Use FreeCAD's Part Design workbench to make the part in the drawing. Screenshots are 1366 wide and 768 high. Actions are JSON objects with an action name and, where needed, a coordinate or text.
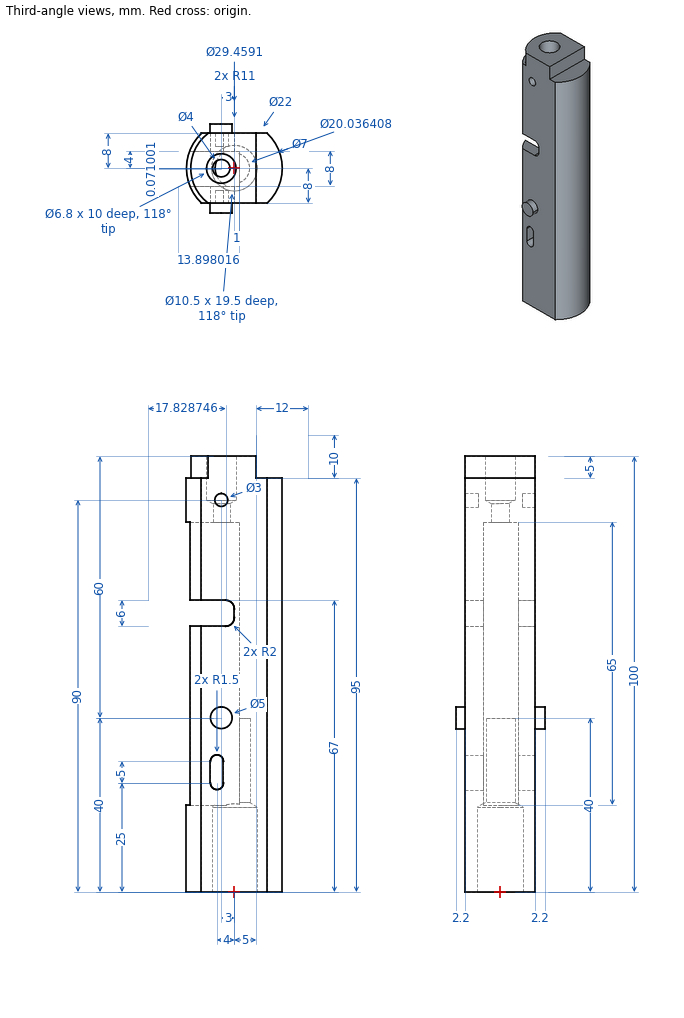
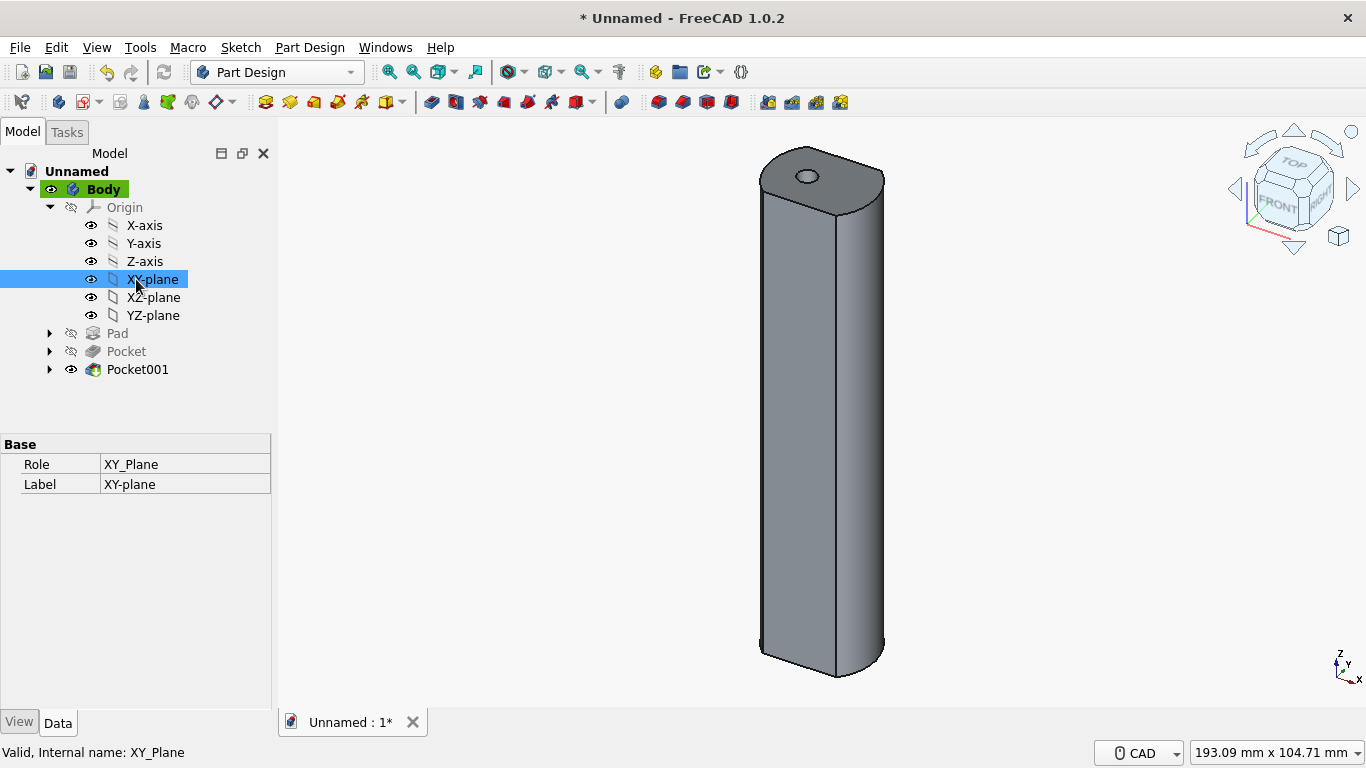
{"action": "left_click", "coordinate": [216, 102]}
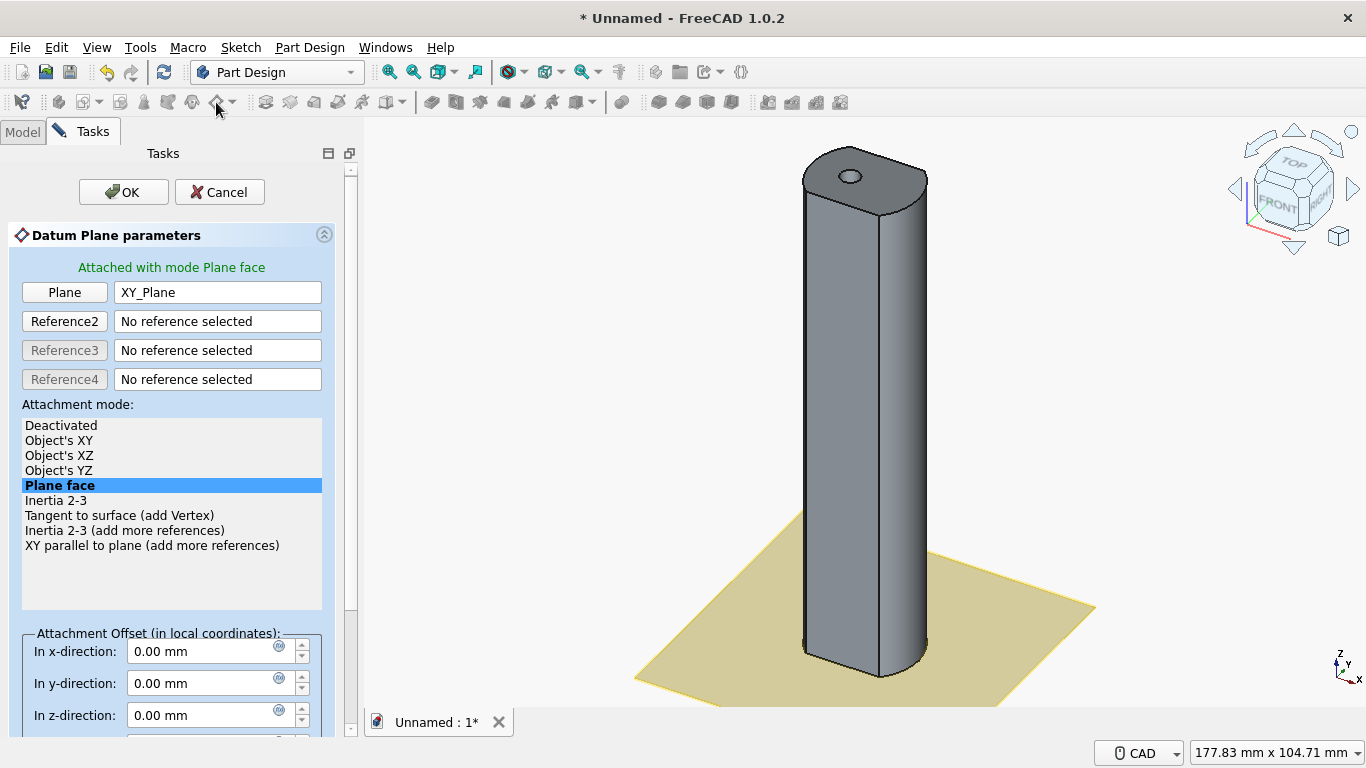
{"action": "triple_click", "coordinate": [210, 715]}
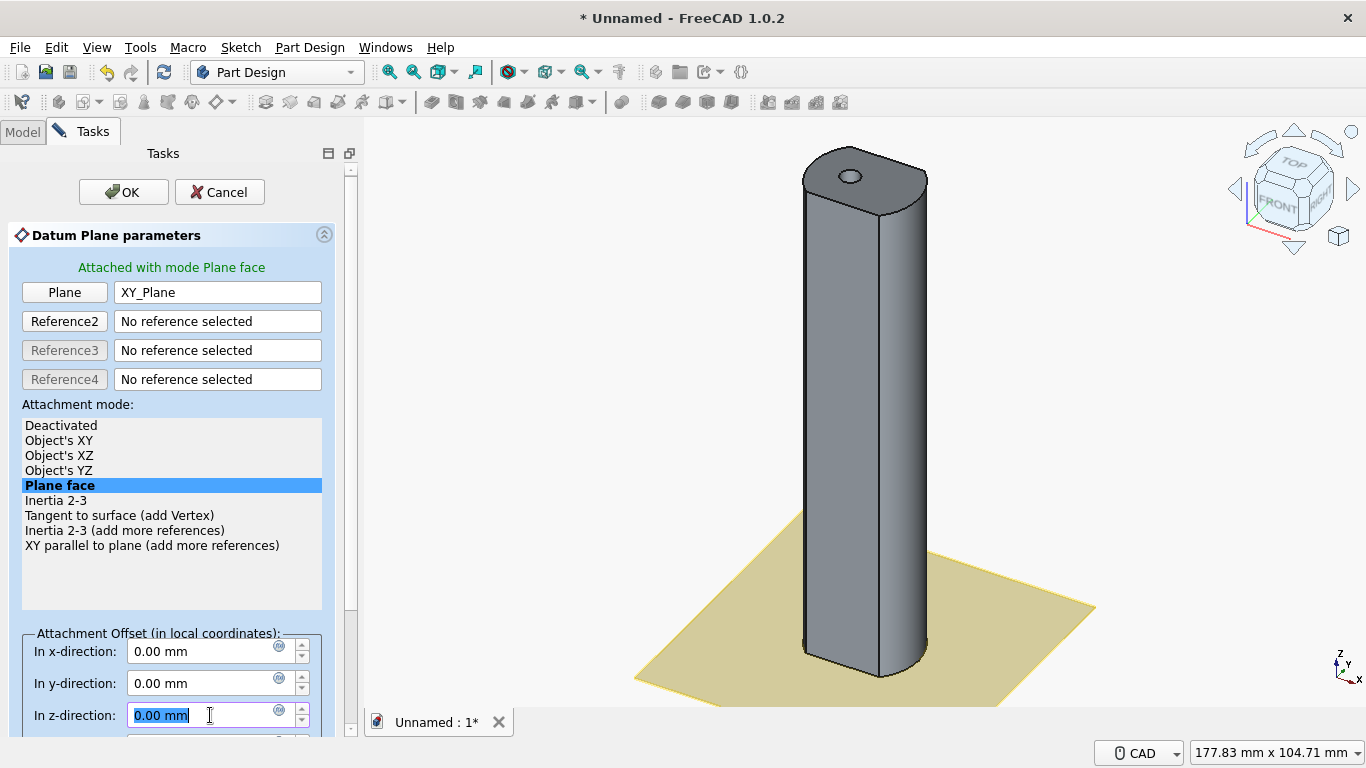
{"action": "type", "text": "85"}
{"action": "key", "text": "Tab"}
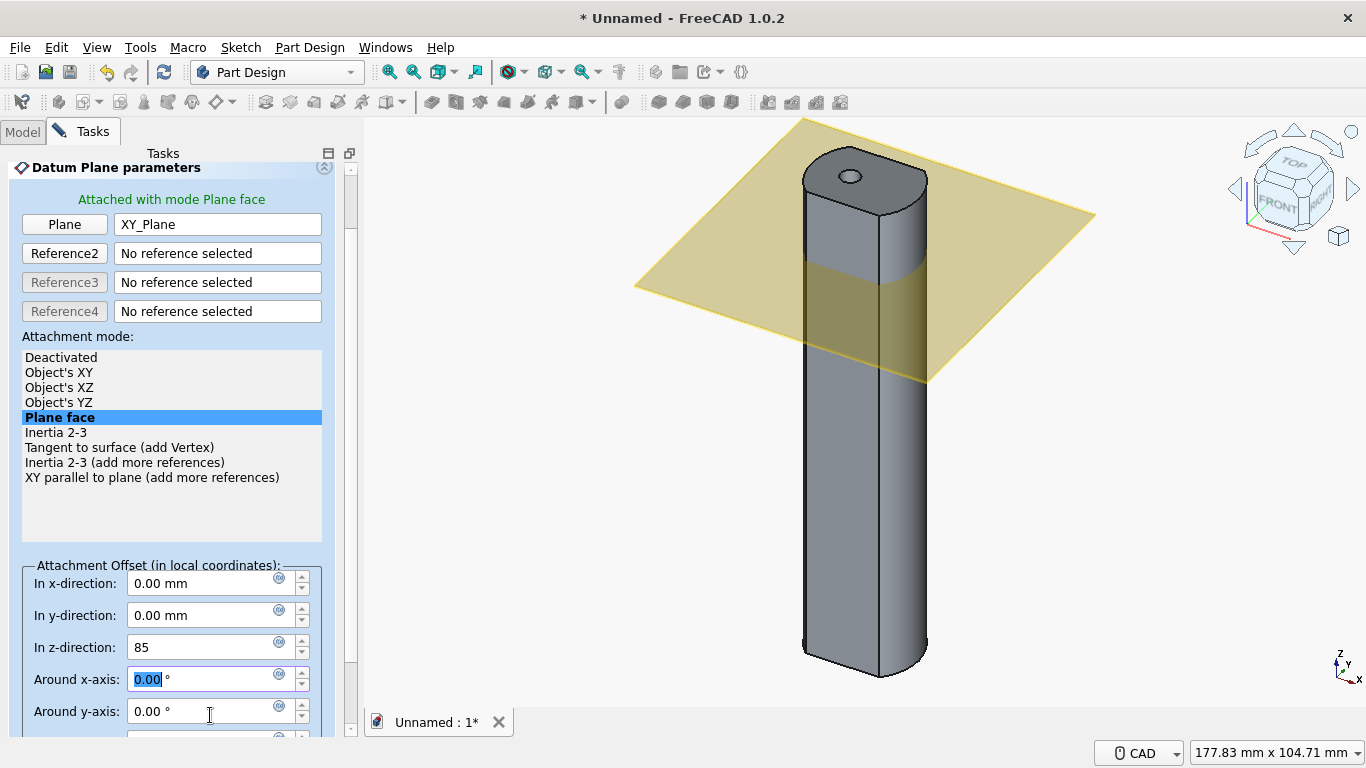
{"action": "scroll", "coordinate": [351, 450], "scroll_direction": "up", "scroll_amount": 2}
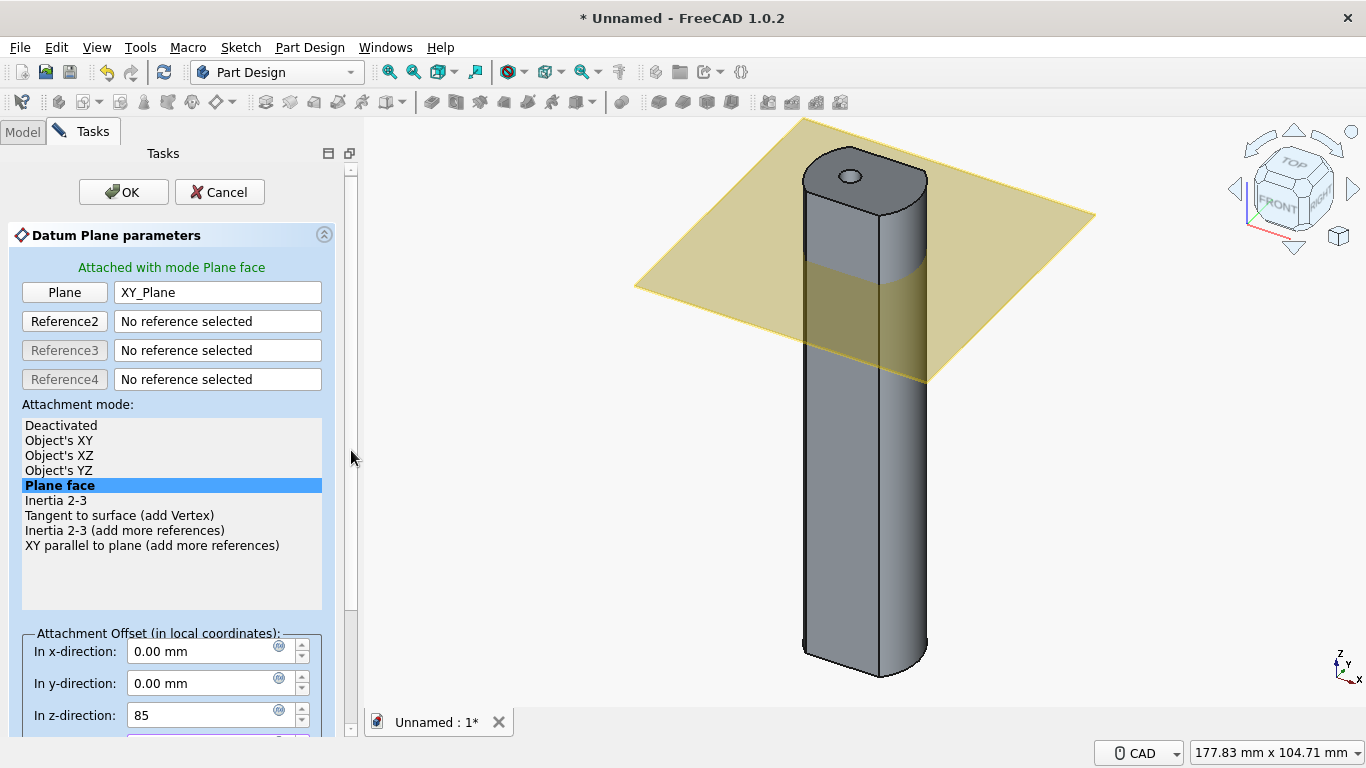
{"action": "left_click", "coordinate": [124, 192]}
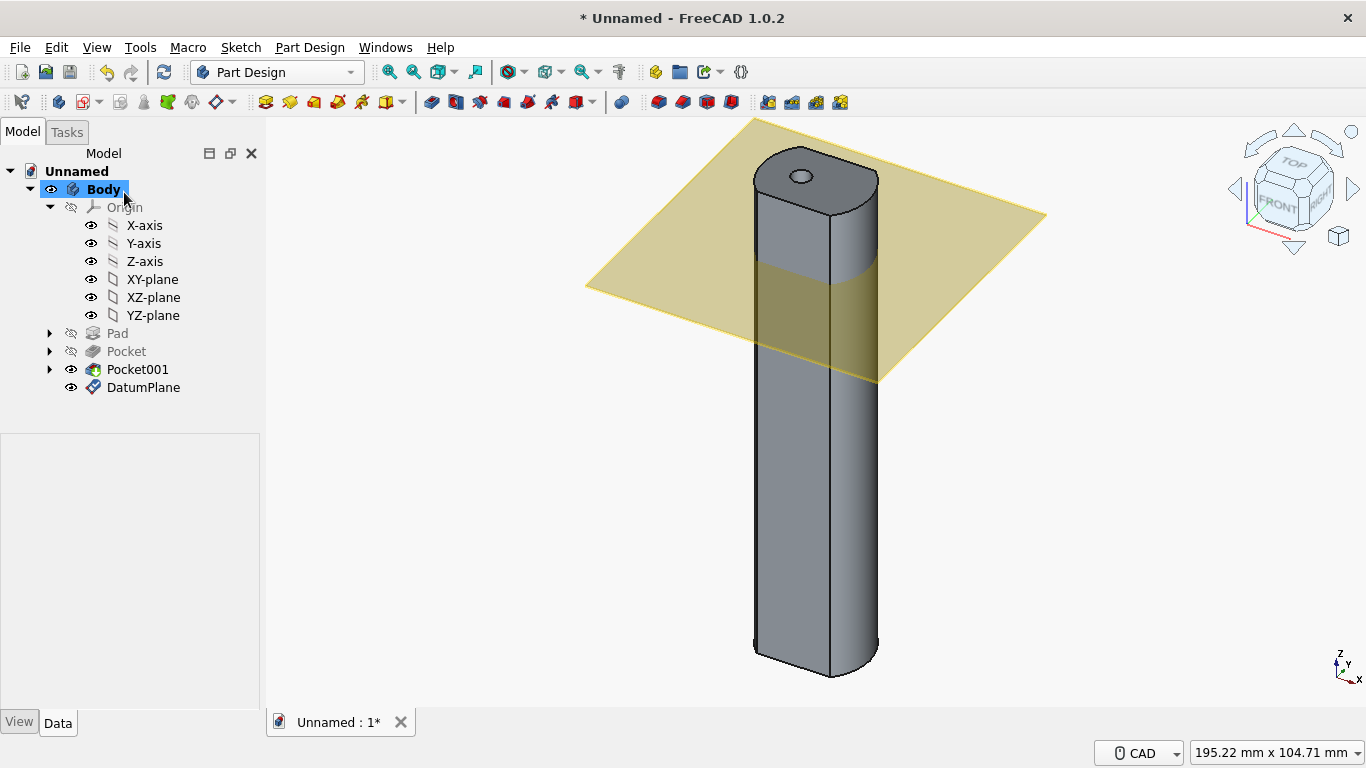
{"action": "left_click", "coordinate": [116, 387]}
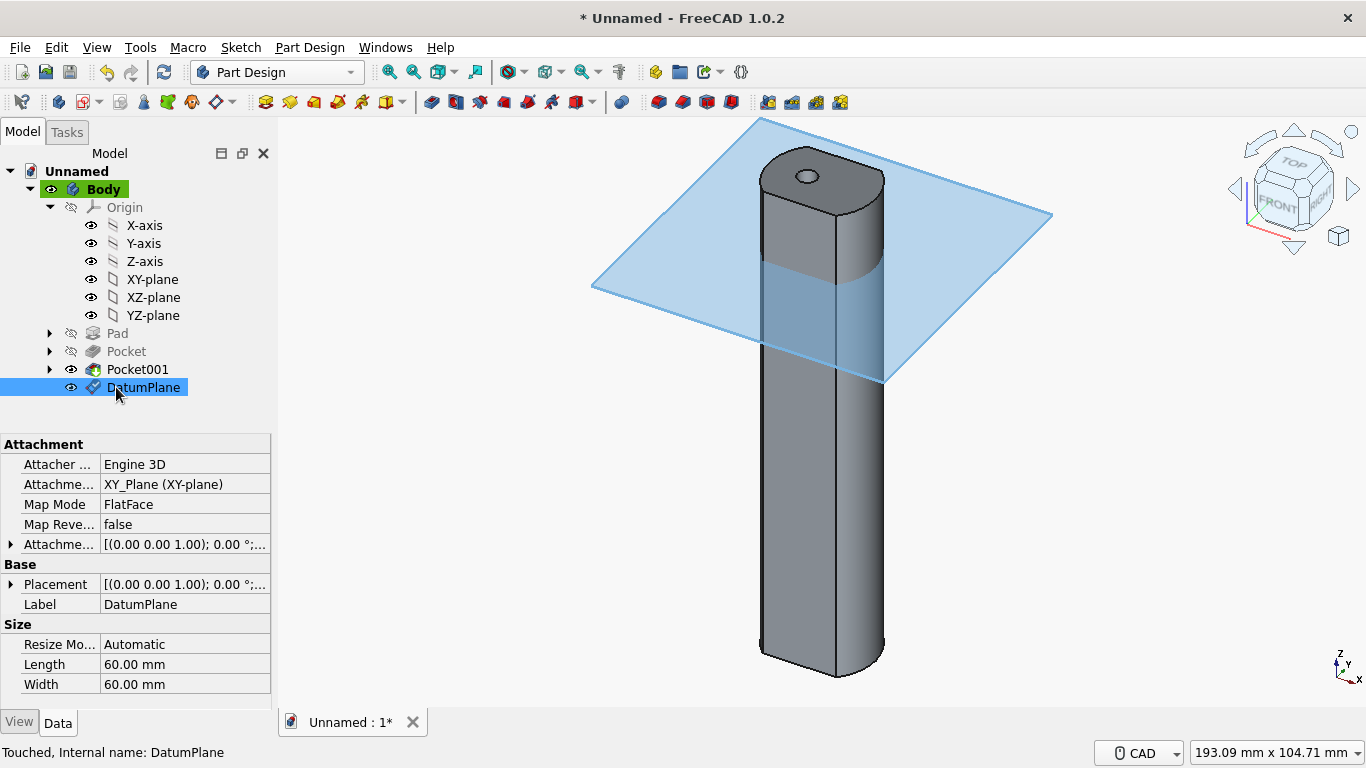
{"action": "left_click", "coordinate": [84, 102]}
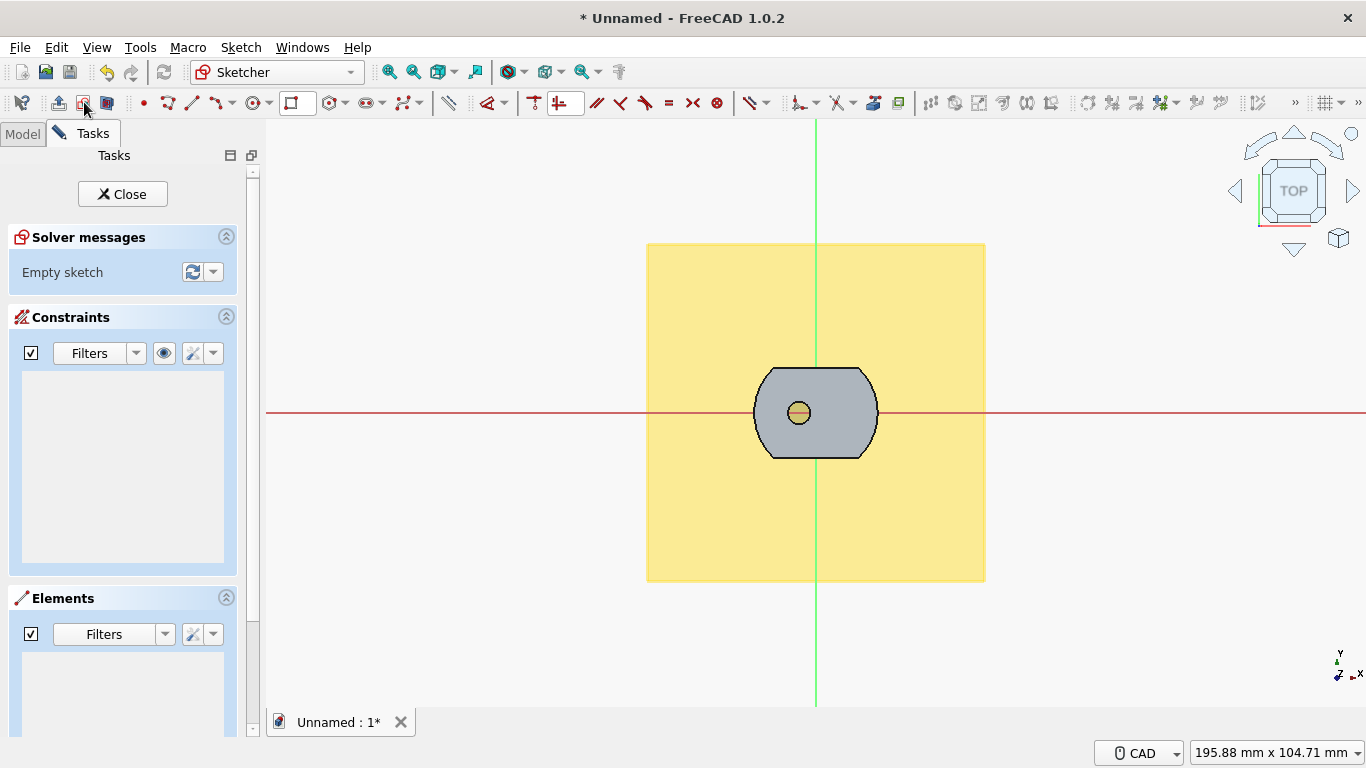
{"action": "left_click", "coordinate": [108, 104]}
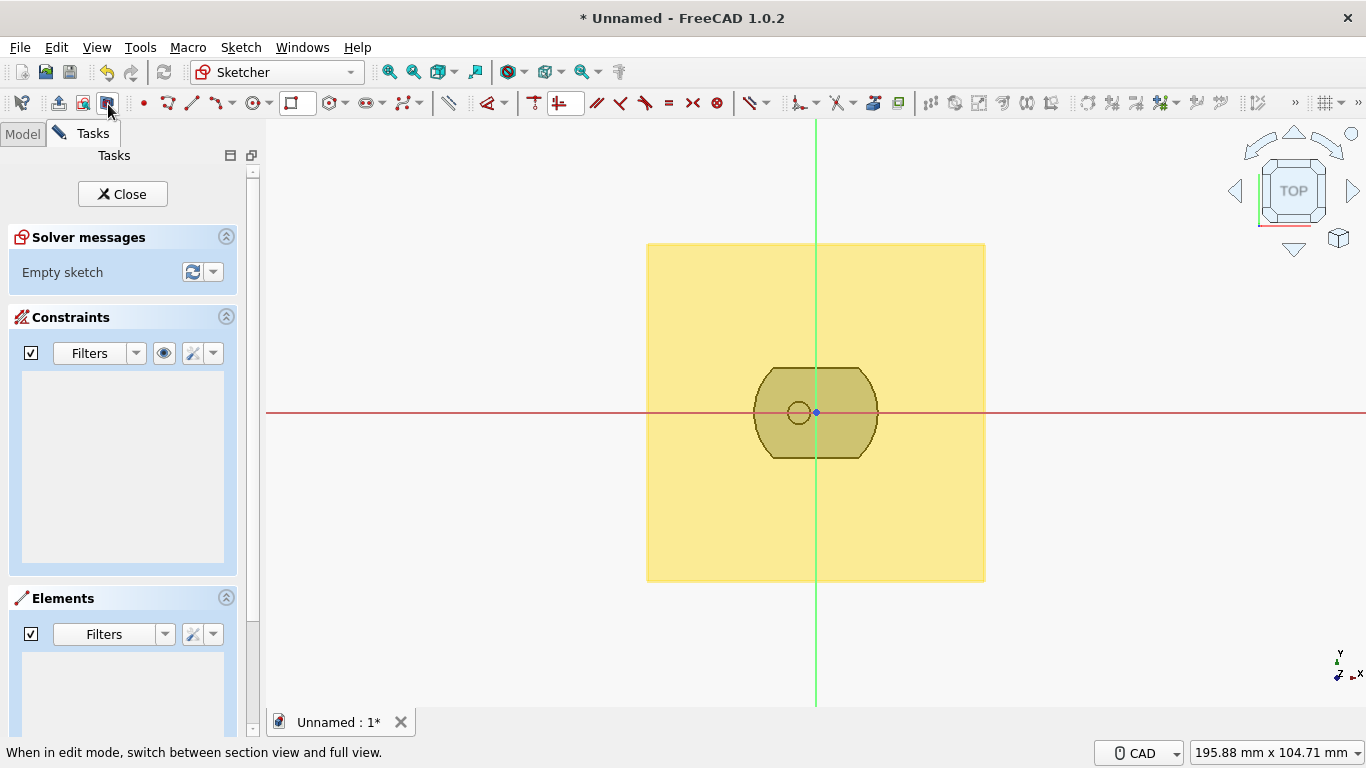
{"action": "scroll", "coordinate": [787, 413], "scroll_direction": "up", "scroll_amount": 11}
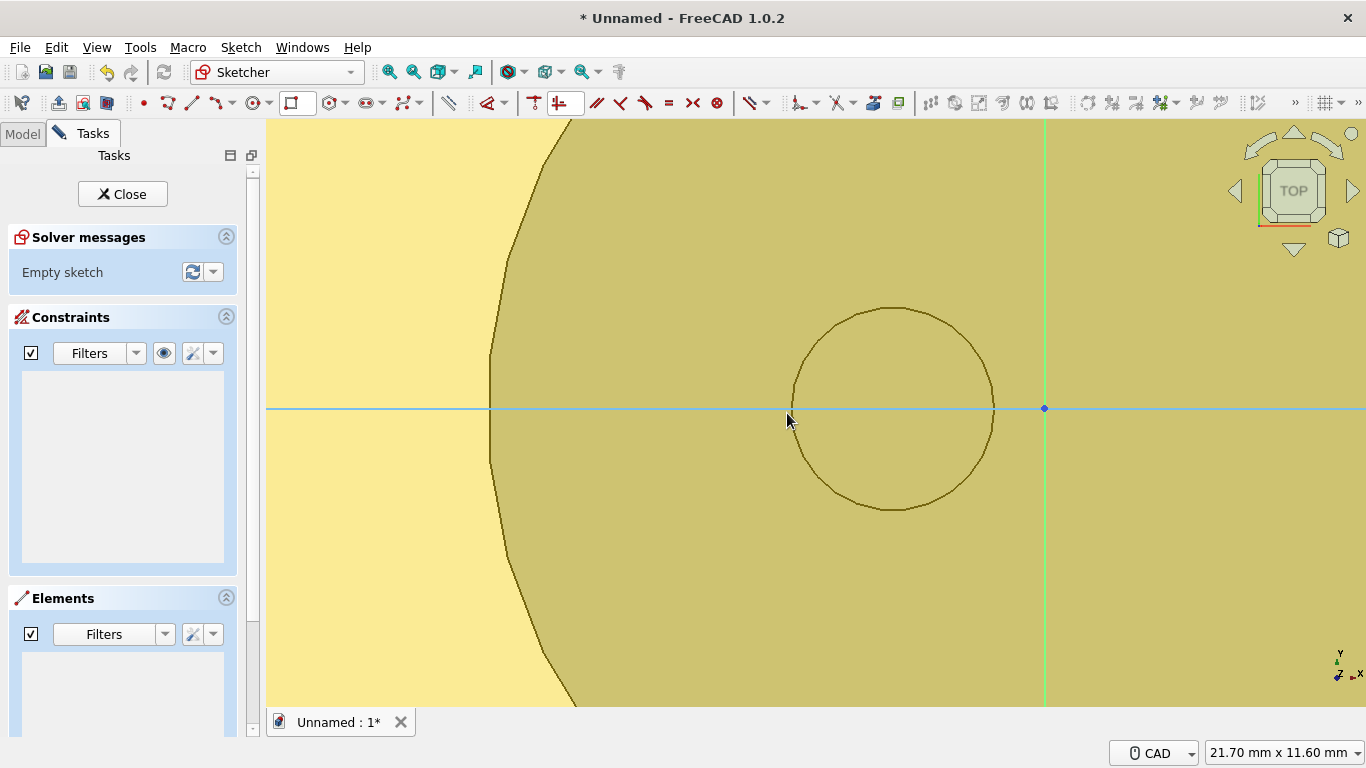
{"action": "key", "text": "g r"}